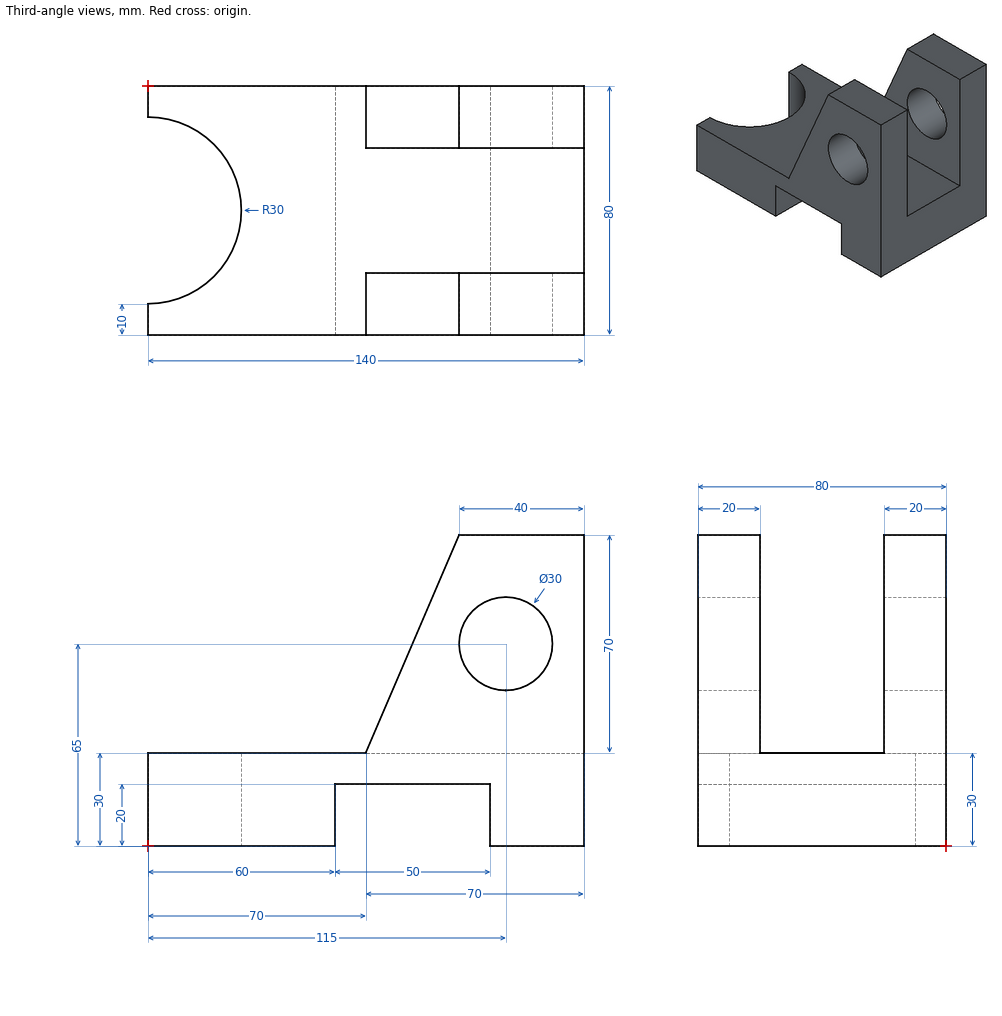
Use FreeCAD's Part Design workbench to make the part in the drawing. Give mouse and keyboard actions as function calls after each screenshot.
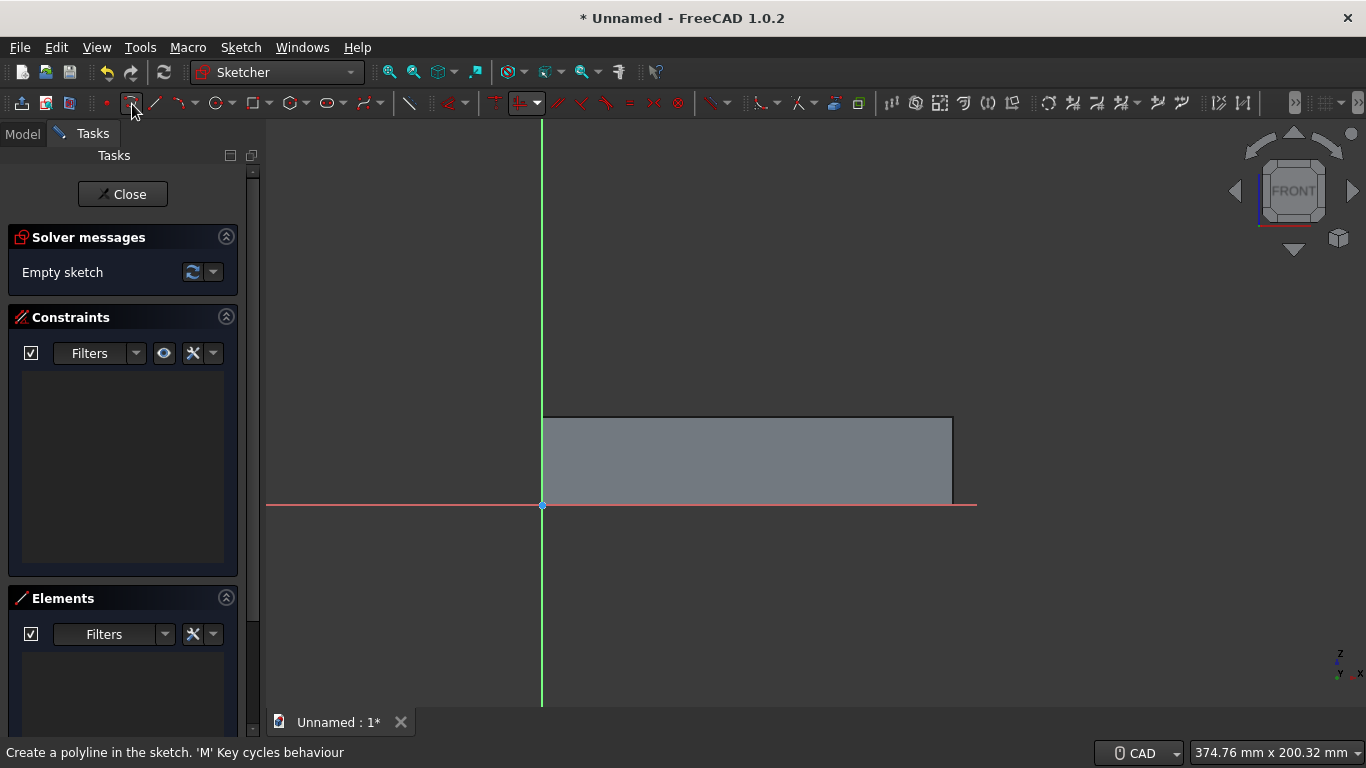
click(748, 417)
click(953, 417)
click(953, 212)
click(836, 212)
click(748, 418)
key(Escape)
key(Escape)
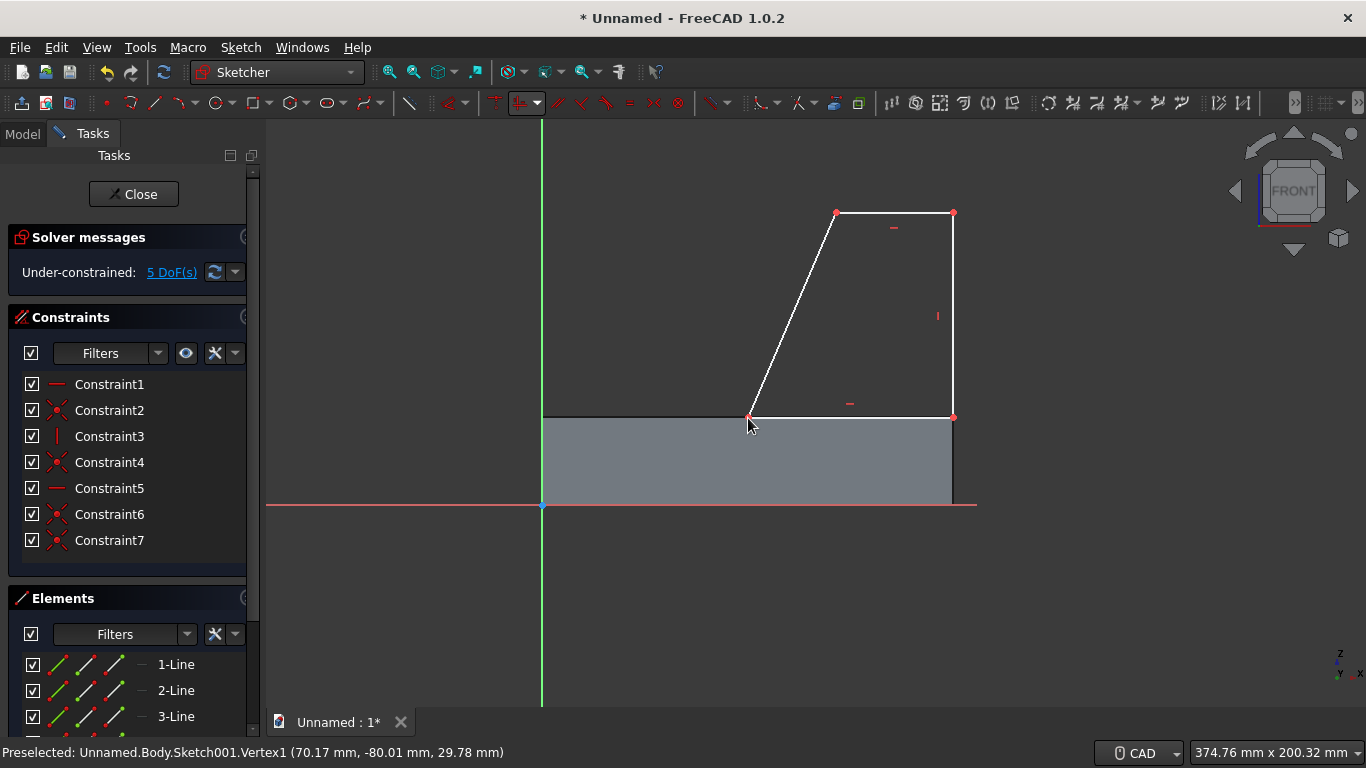
click(448, 104)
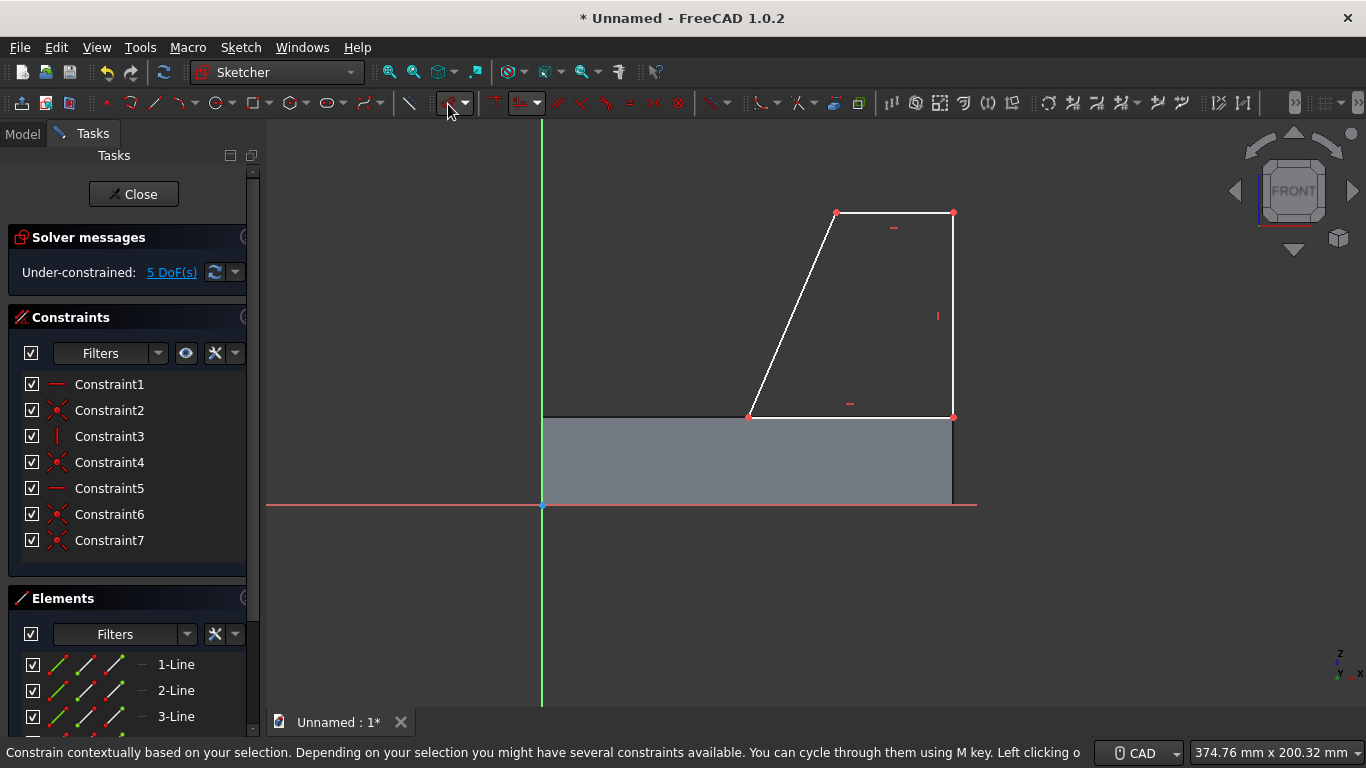
click(810, 418)
click(851, 452)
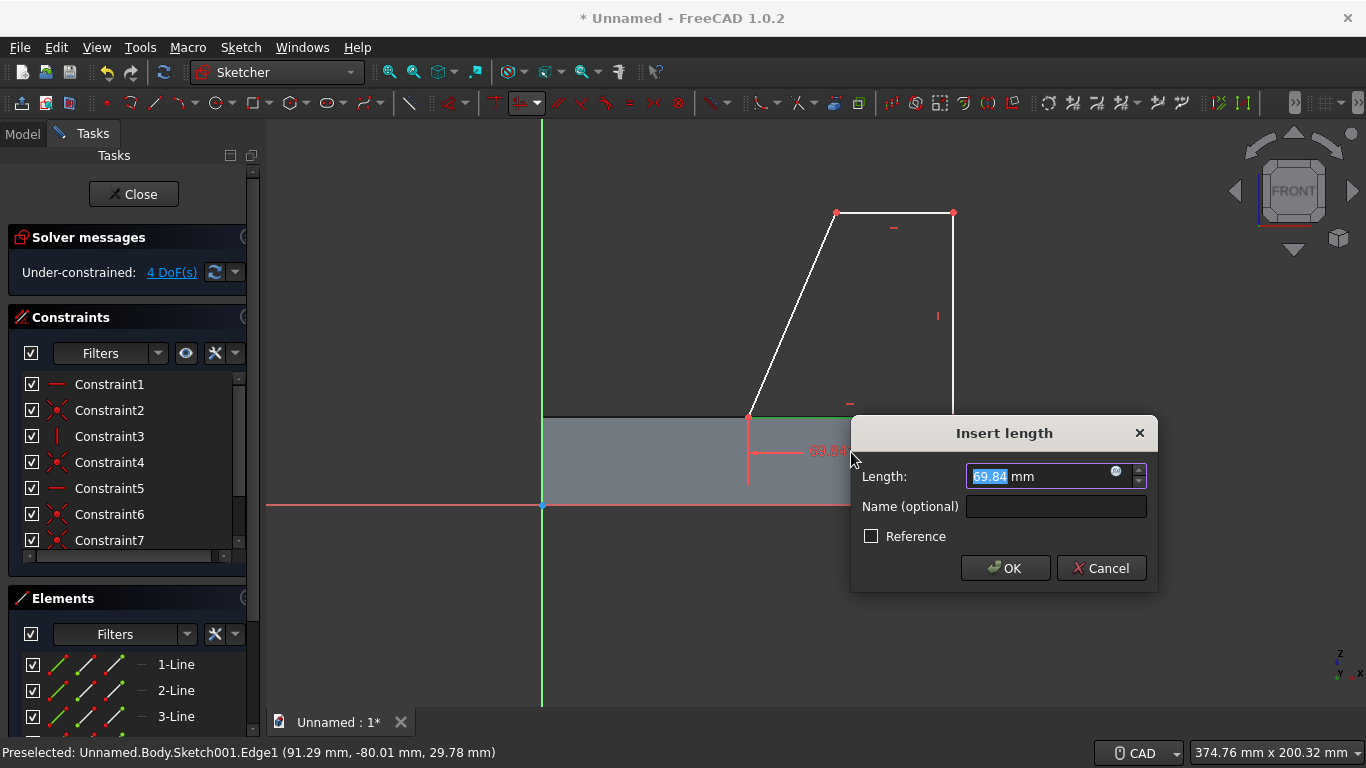
text(70)
key(Return)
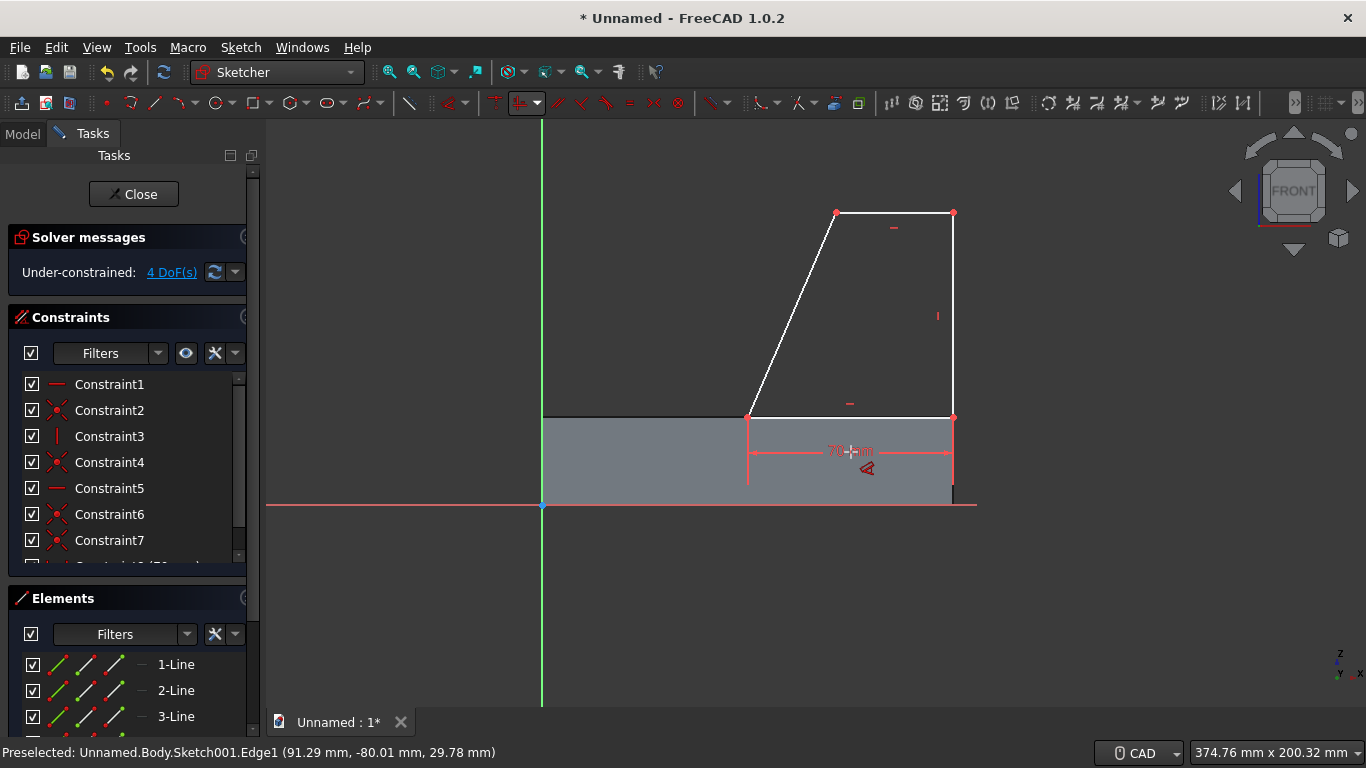
click(953, 357)
click(987, 315)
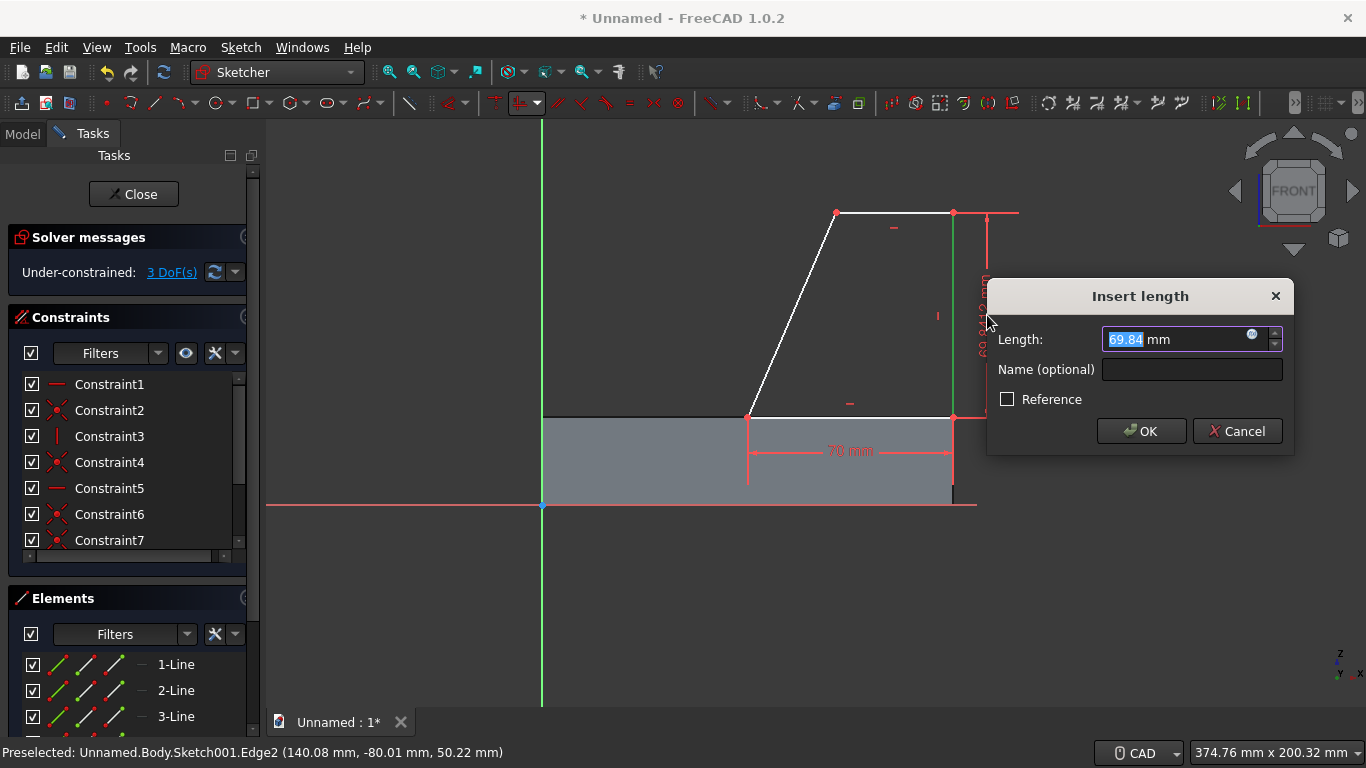
text(70)
key(Return)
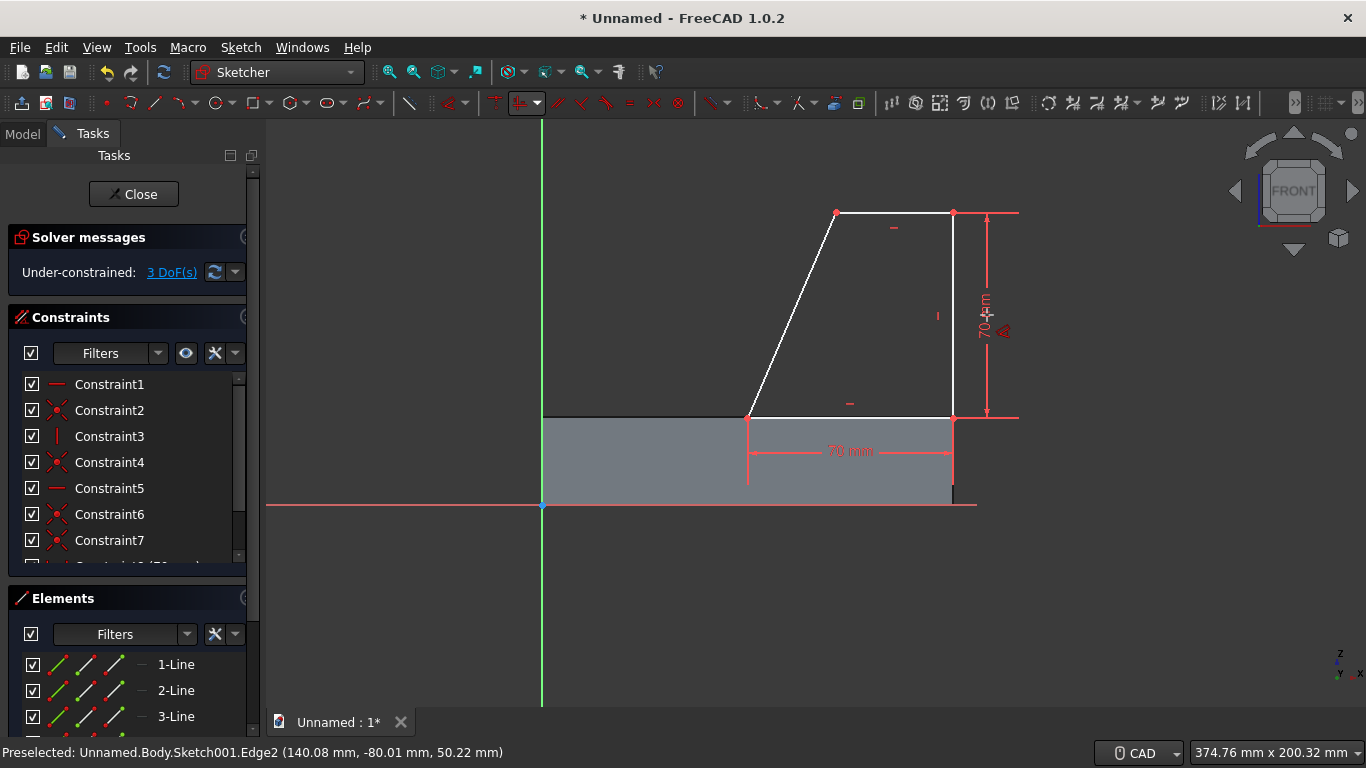
click(918, 213)
click(895, 179)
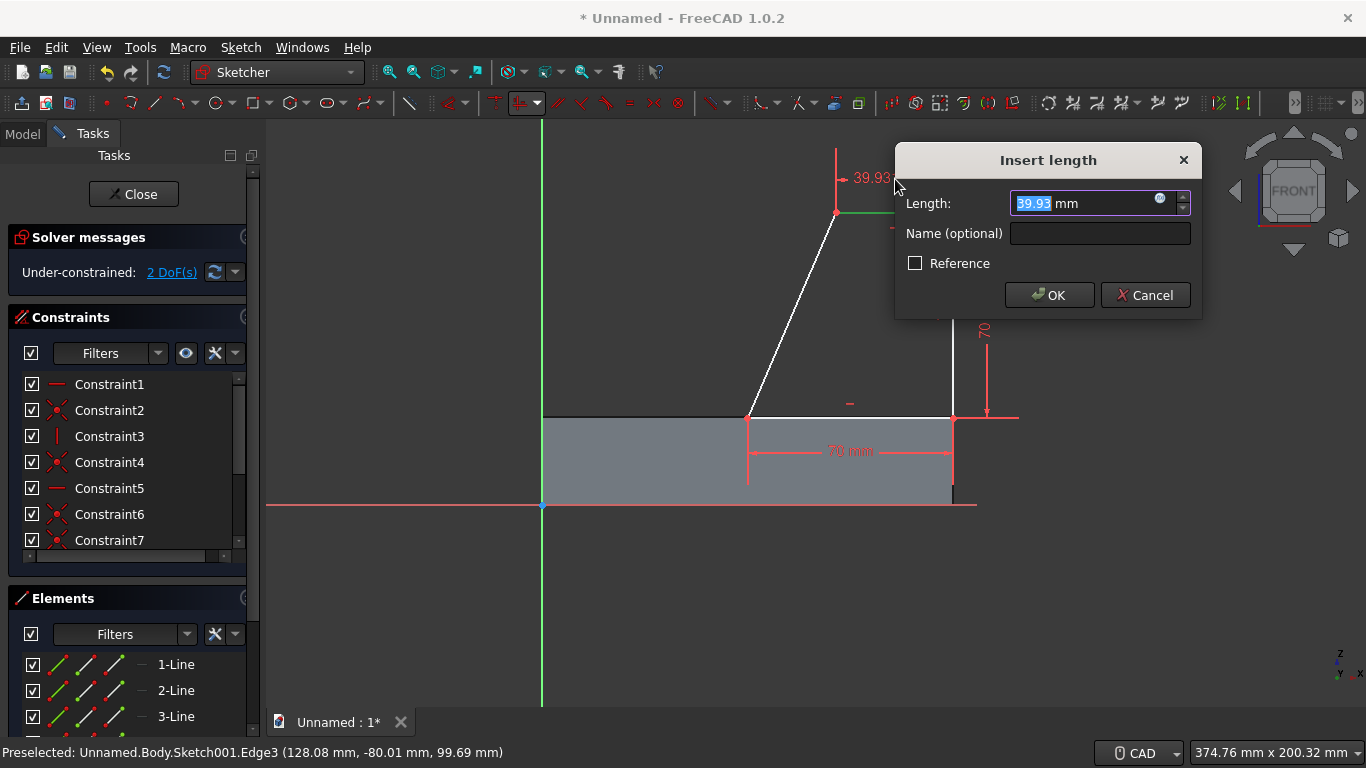
text(40)
key(Return)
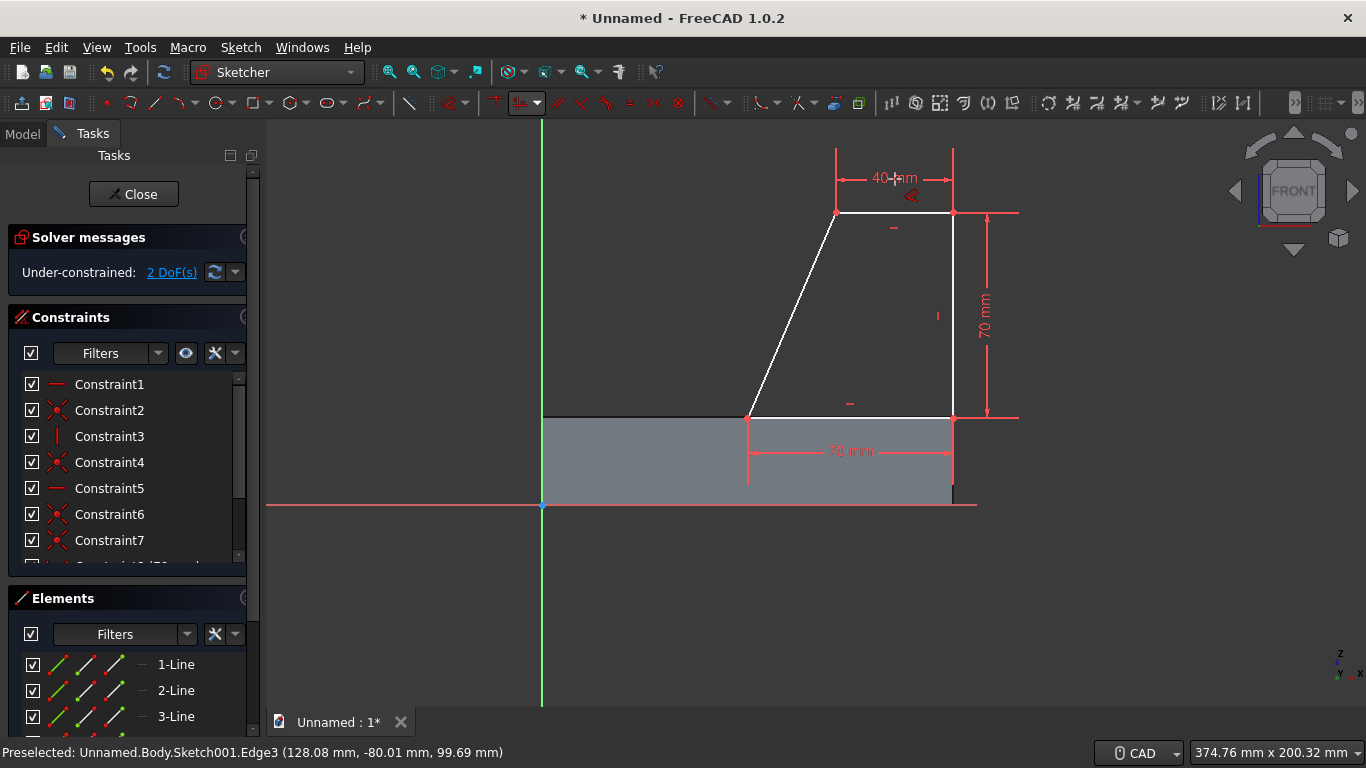
click(748, 418)
click(645, 539)